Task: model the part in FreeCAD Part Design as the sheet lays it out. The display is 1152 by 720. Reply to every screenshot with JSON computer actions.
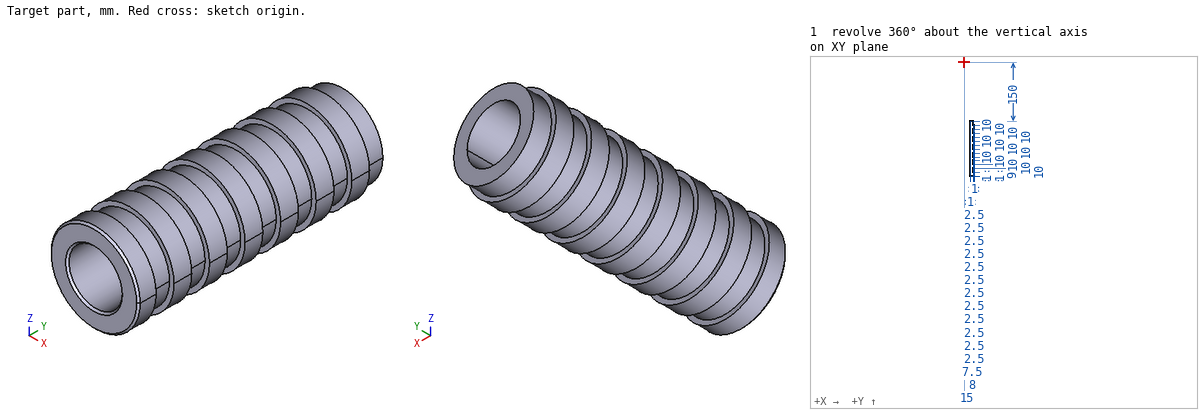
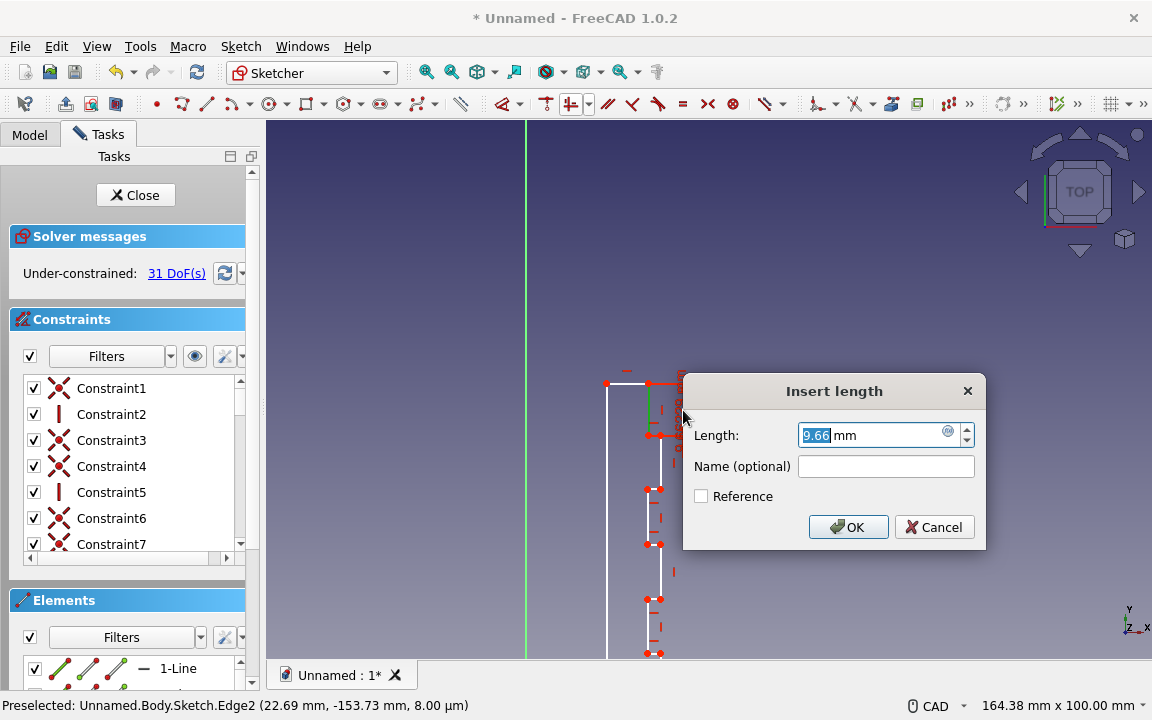
{"action": "type", "text": "10"}
{"action": "key", "text": "Return"}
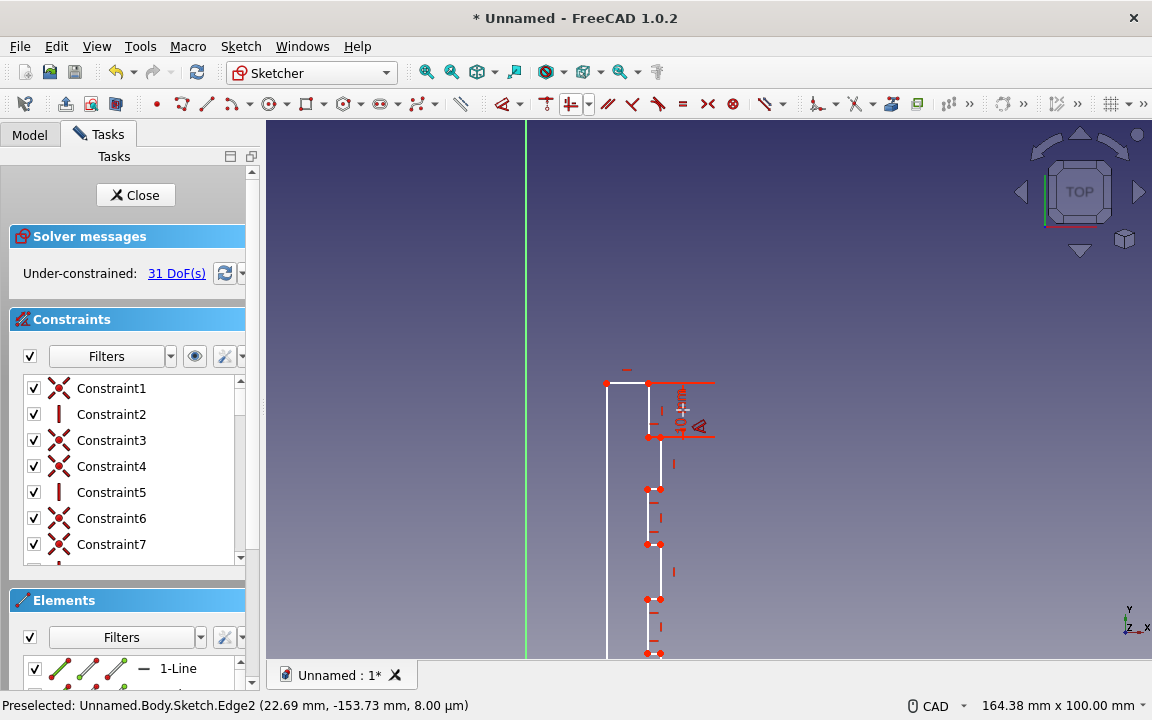
{"action": "left_click", "coordinate": [661, 453]}
{"action": "left_click", "coordinate": [695, 463]}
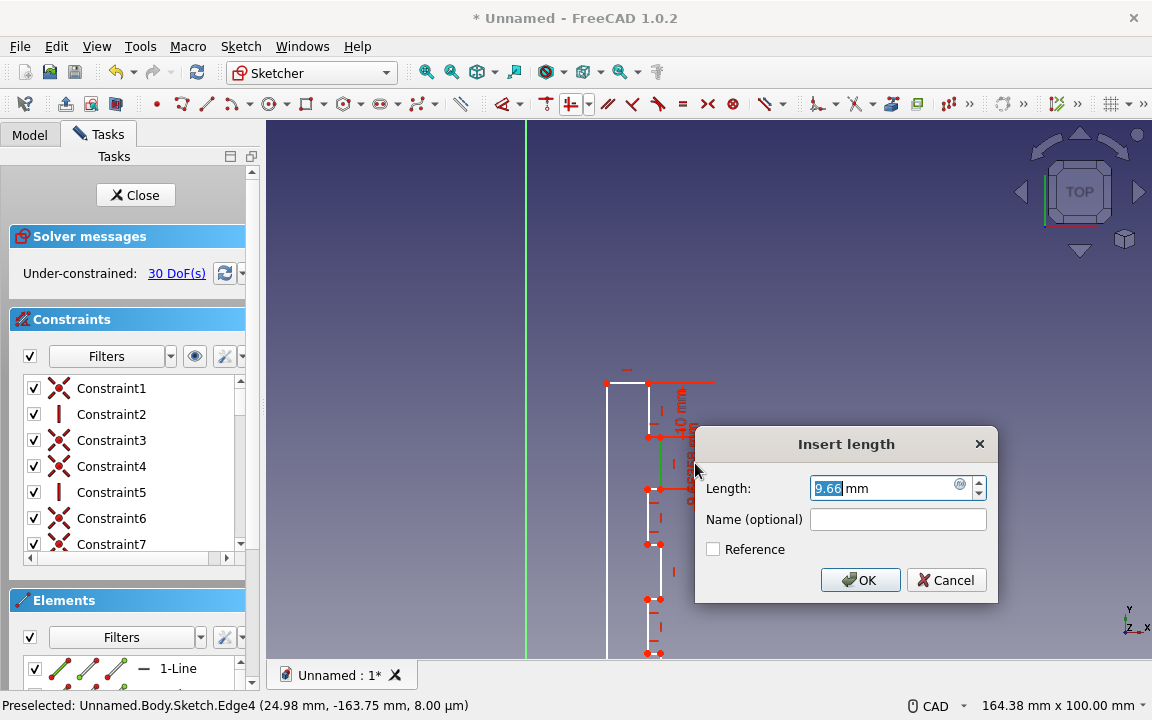
{"action": "type", "text": "10"}
{"action": "key", "text": "Return"}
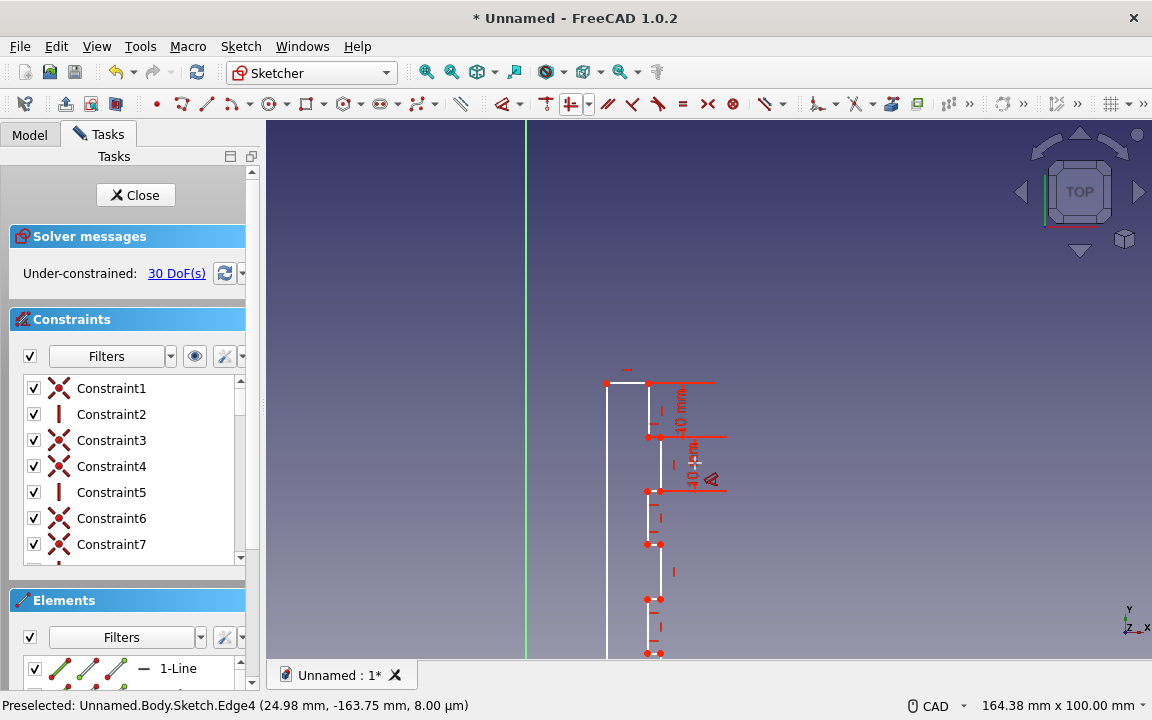
{"action": "left_click", "coordinate": [648, 507]}
{"action": "left_click", "coordinate": [682, 518]}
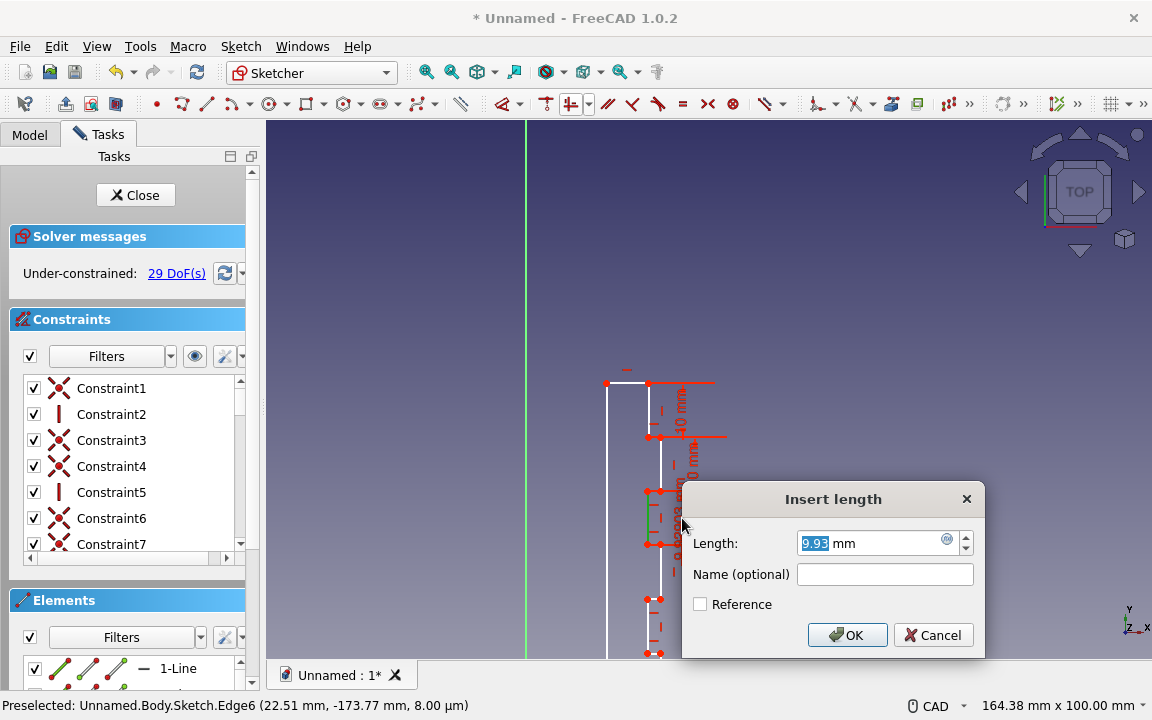
{"action": "type", "text": "10"}
{"action": "key", "text": "Return"}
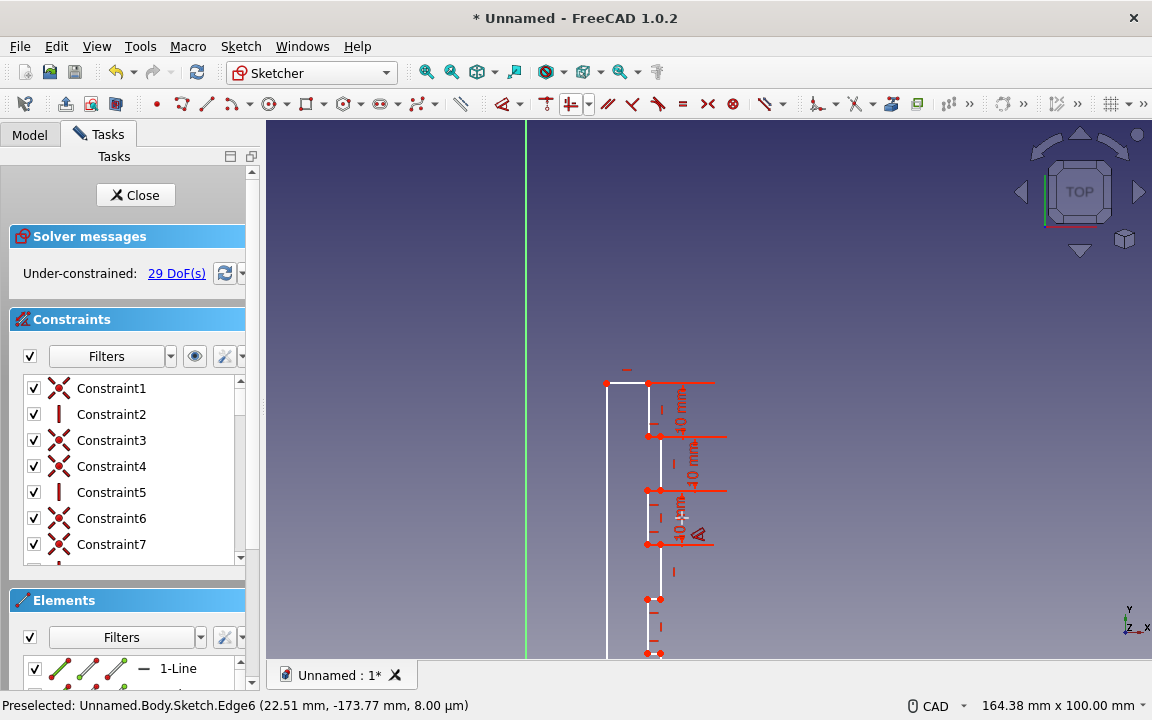
{"action": "left_click", "coordinate": [661, 561]}
{"action": "left_click", "coordinate": [695, 572]}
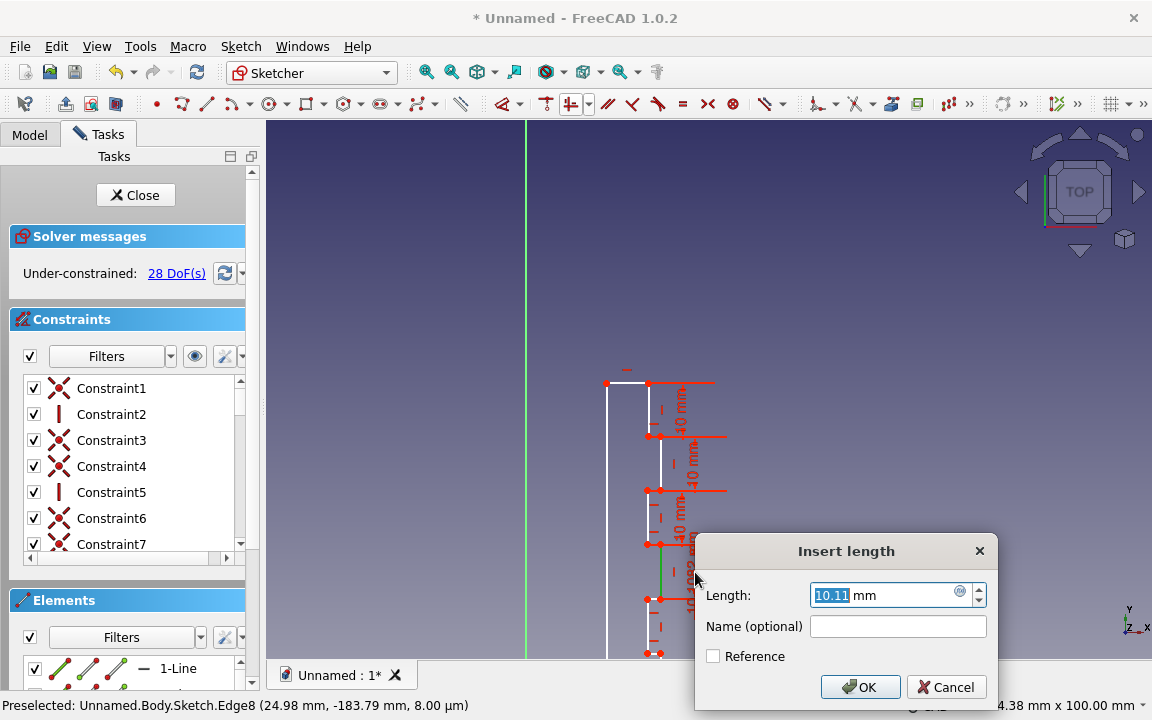
{"action": "type", "text": "10"}
{"action": "key", "text": "Return"}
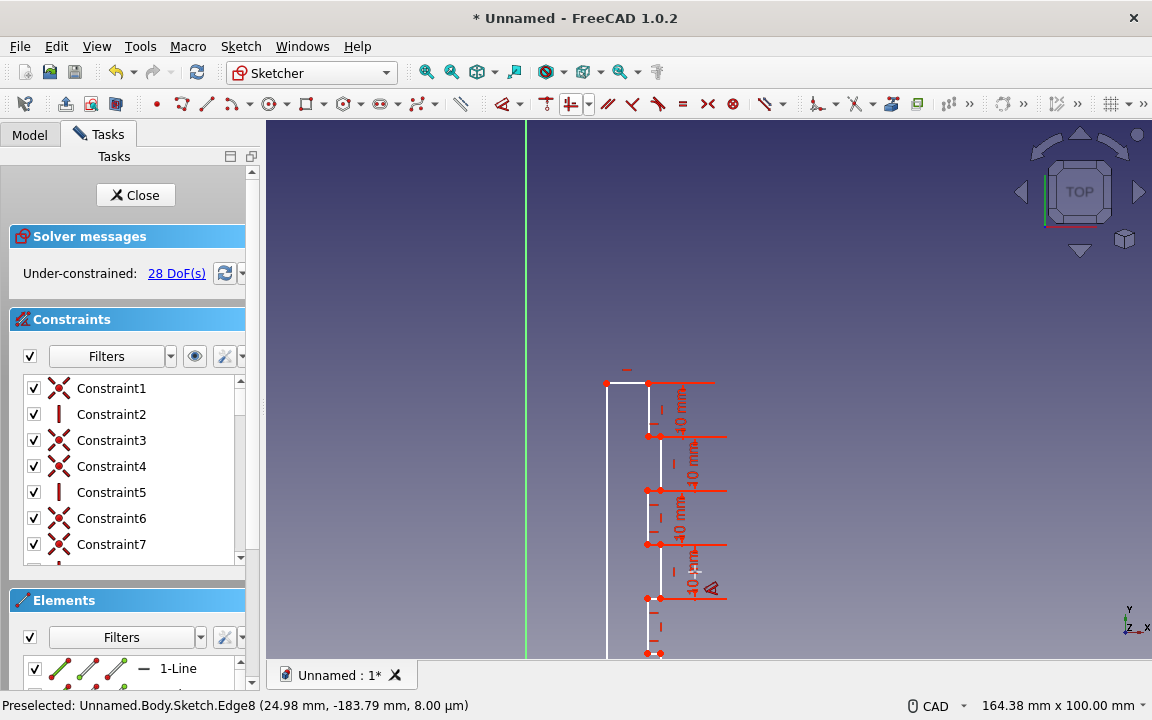
{"action": "left_click", "coordinate": [648, 615]}
{"action": "left_click", "coordinate": [682, 615]}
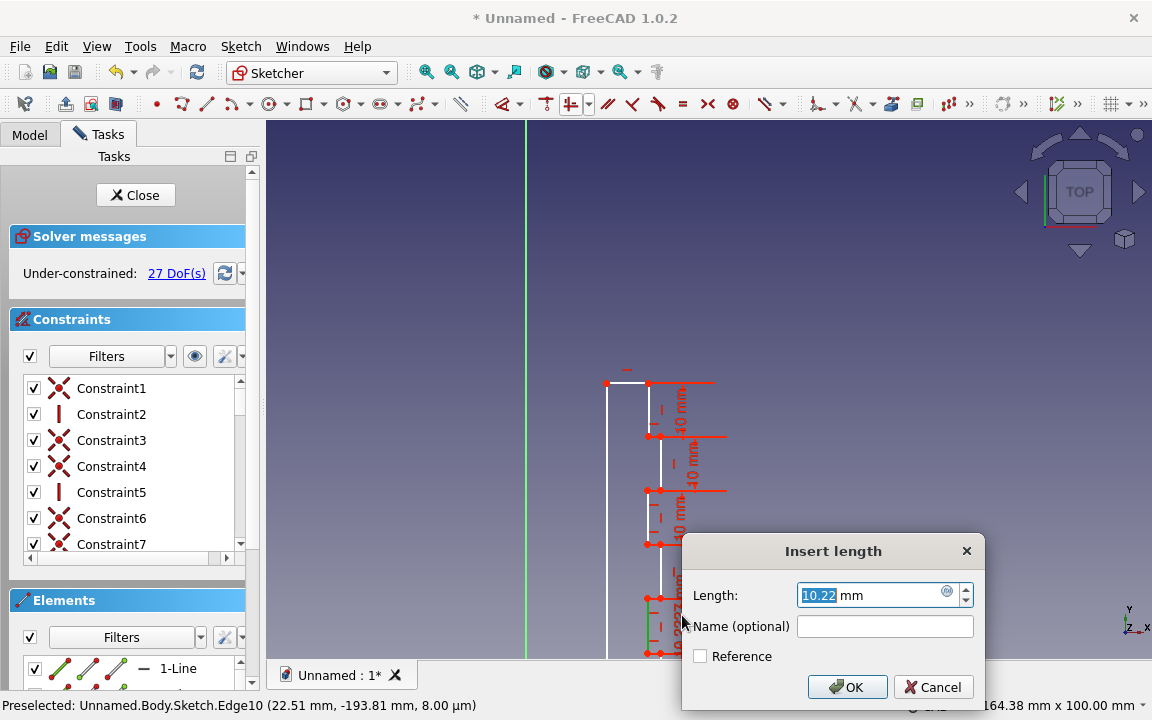
{"action": "type", "text": "10"}
{"action": "key", "text": "Return"}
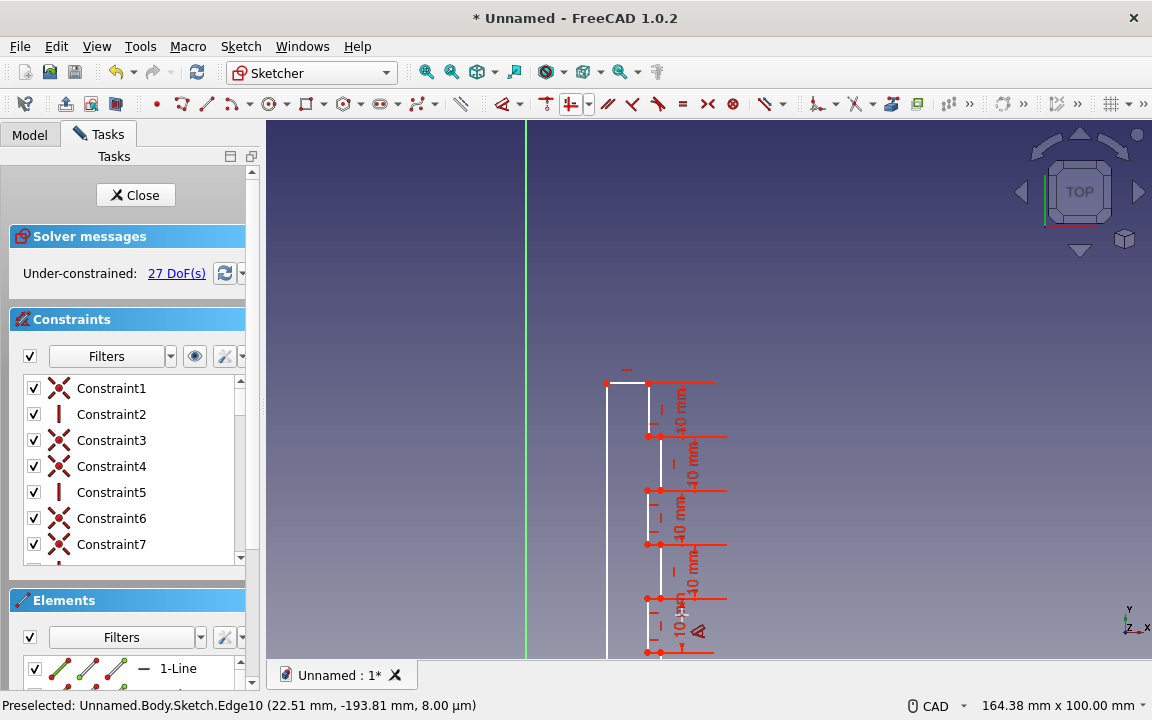
{"action": "scroll", "coordinate": [652, 399], "scroll_direction": "down", "scroll_amount": 8}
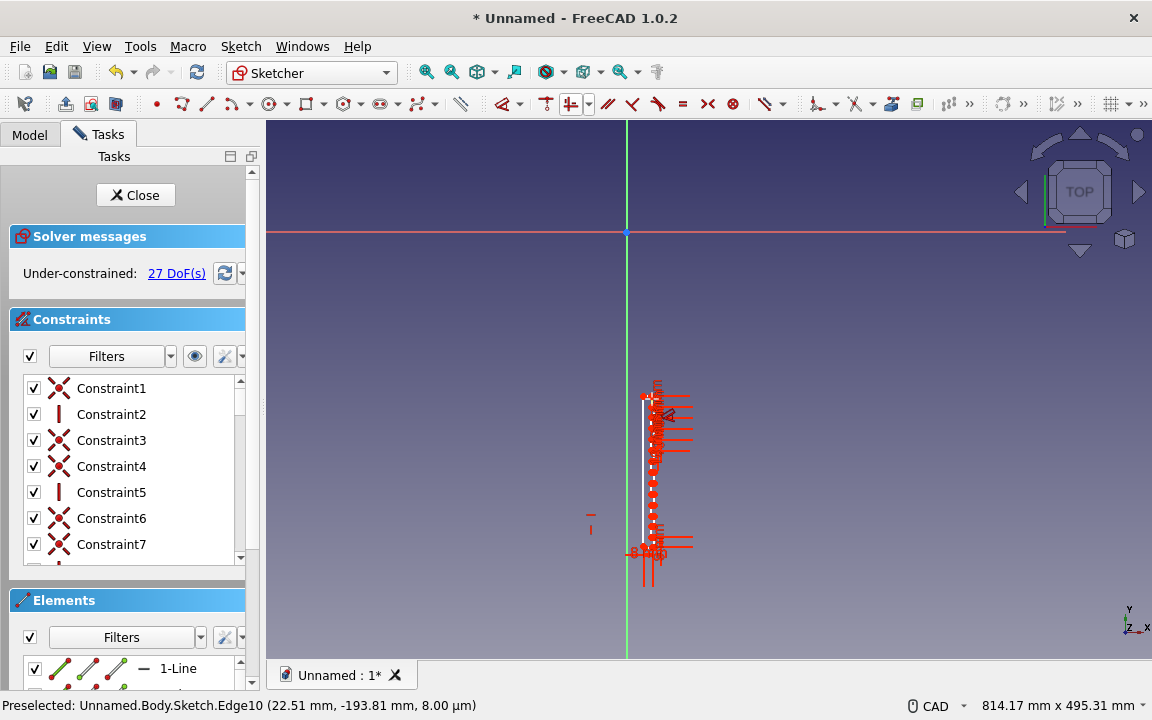
{"action": "scroll", "coordinate": [654, 454], "scroll_direction": "up", "scroll_amount": 8}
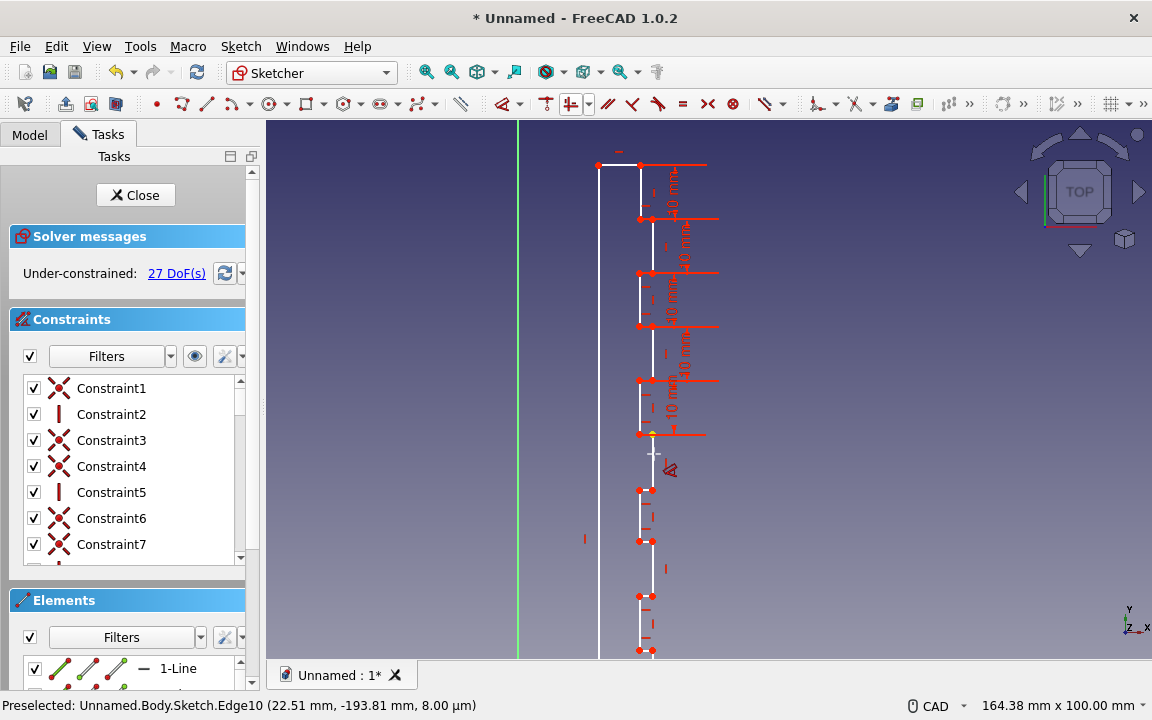
{"action": "left_click", "coordinate": [653, 451]}
{"action": "left_click", "coordinate": [687, 463]}